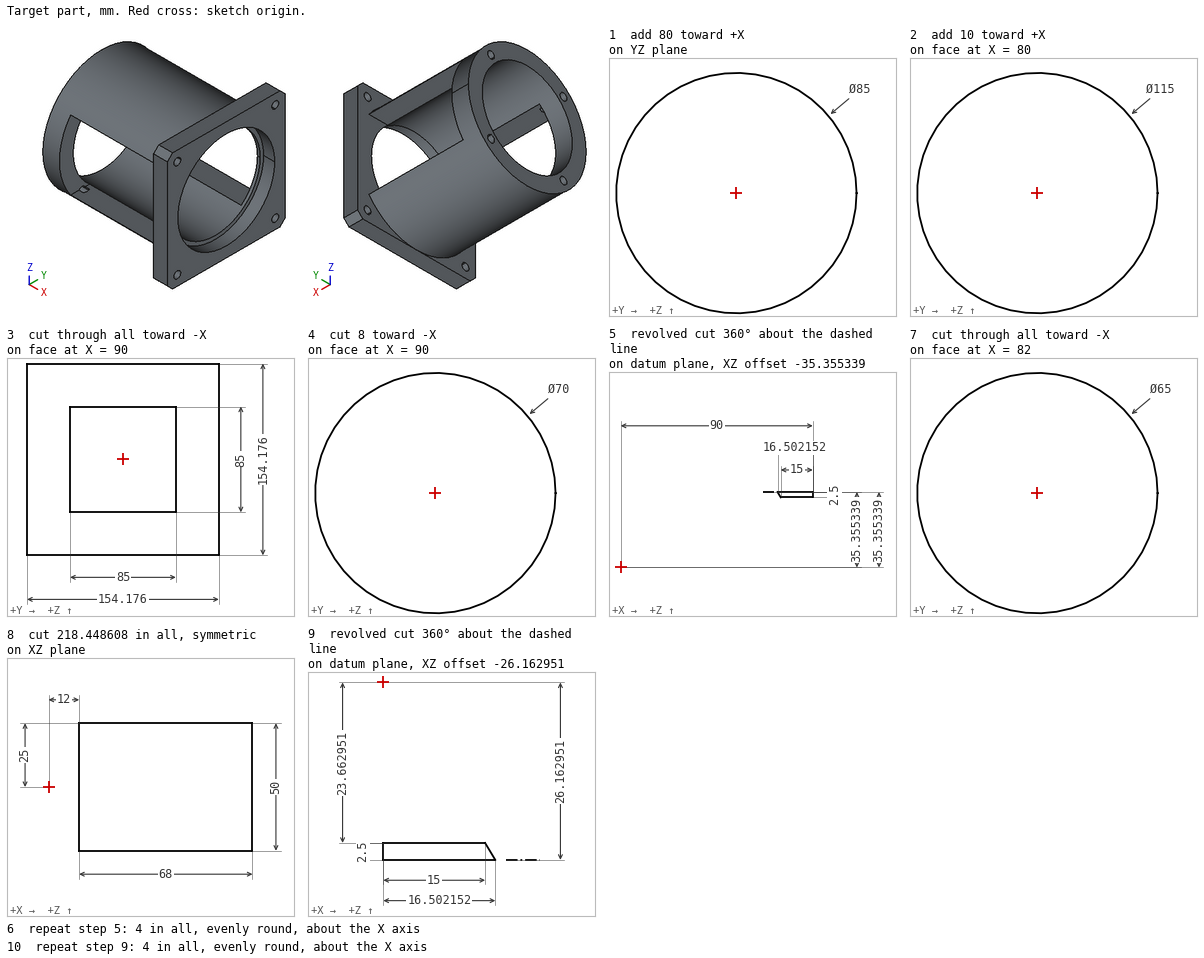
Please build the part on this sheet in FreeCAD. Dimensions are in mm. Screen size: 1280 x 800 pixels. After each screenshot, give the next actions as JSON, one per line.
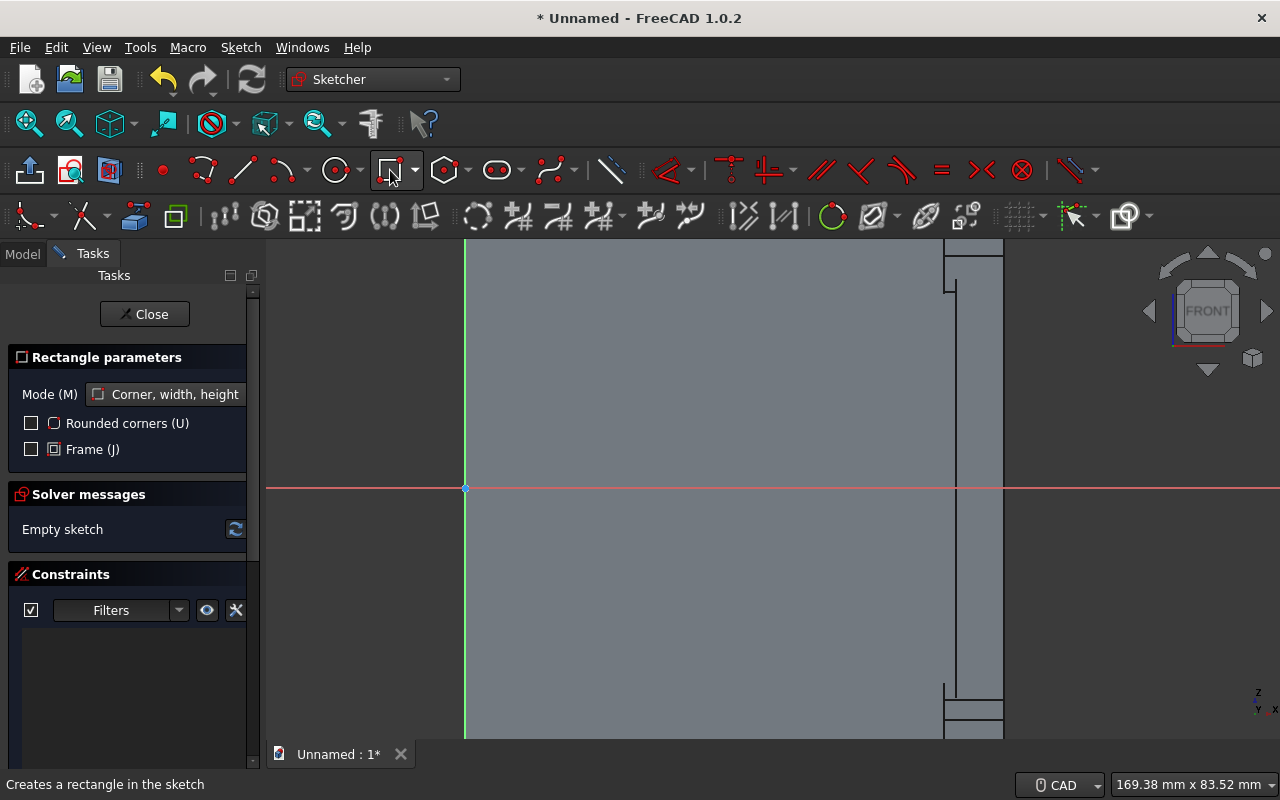
{"action": "left_click", "coordinate": [537, 339]}
{"action": "mouse_move", "coordinate": [944, 638]}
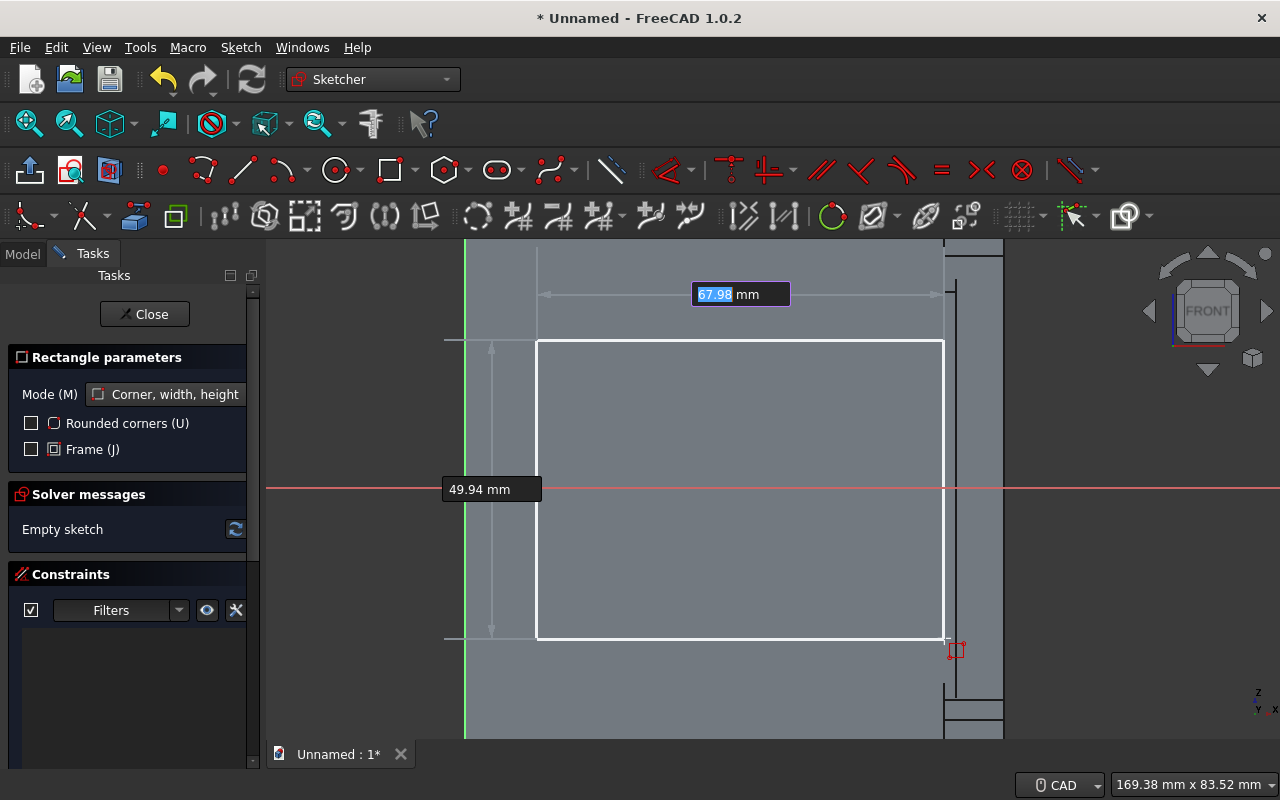
{"action": "type", "text": "68"}
{"action": "key", "text": "Tab"}
{"action": "type", "text": "50"}
{"action": "key", "text": "Return"}
{"action": "key", "text": "Escape"}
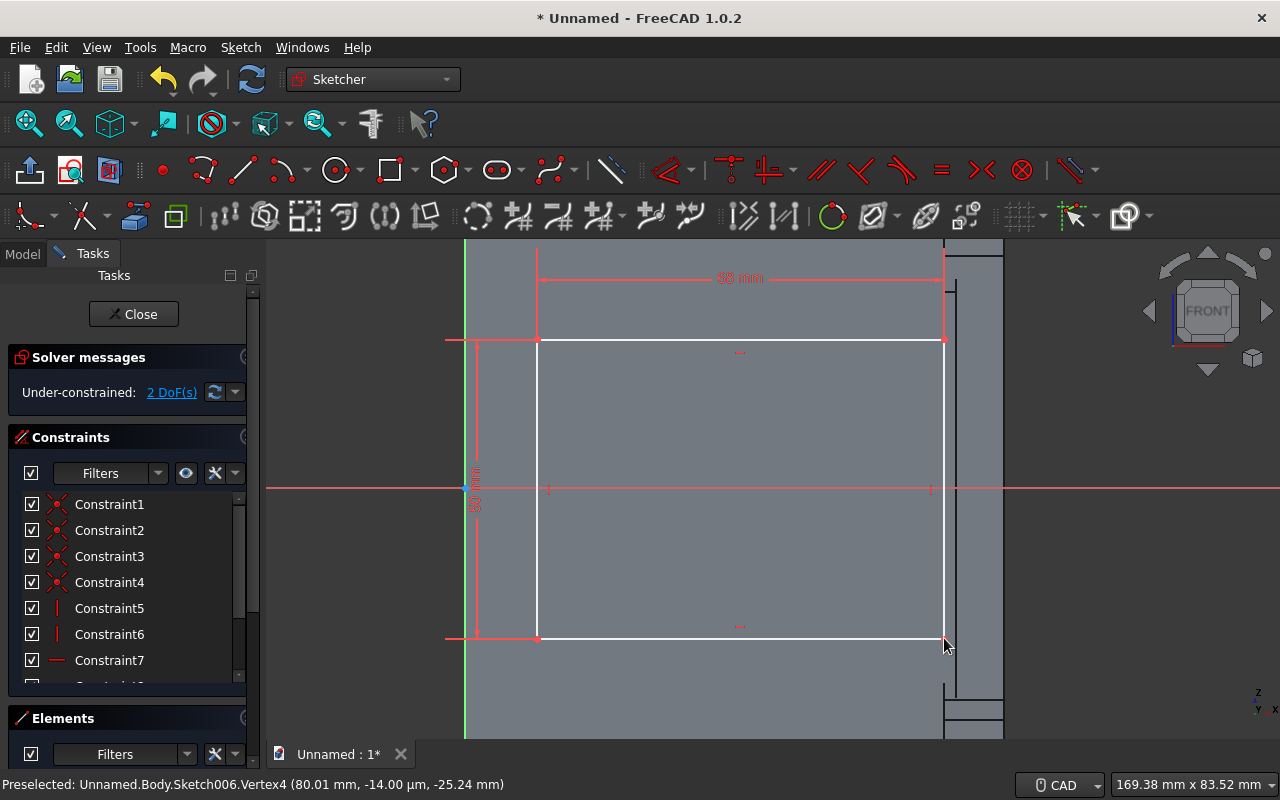
{"action": "left_click", "coordinate": [666, 170]}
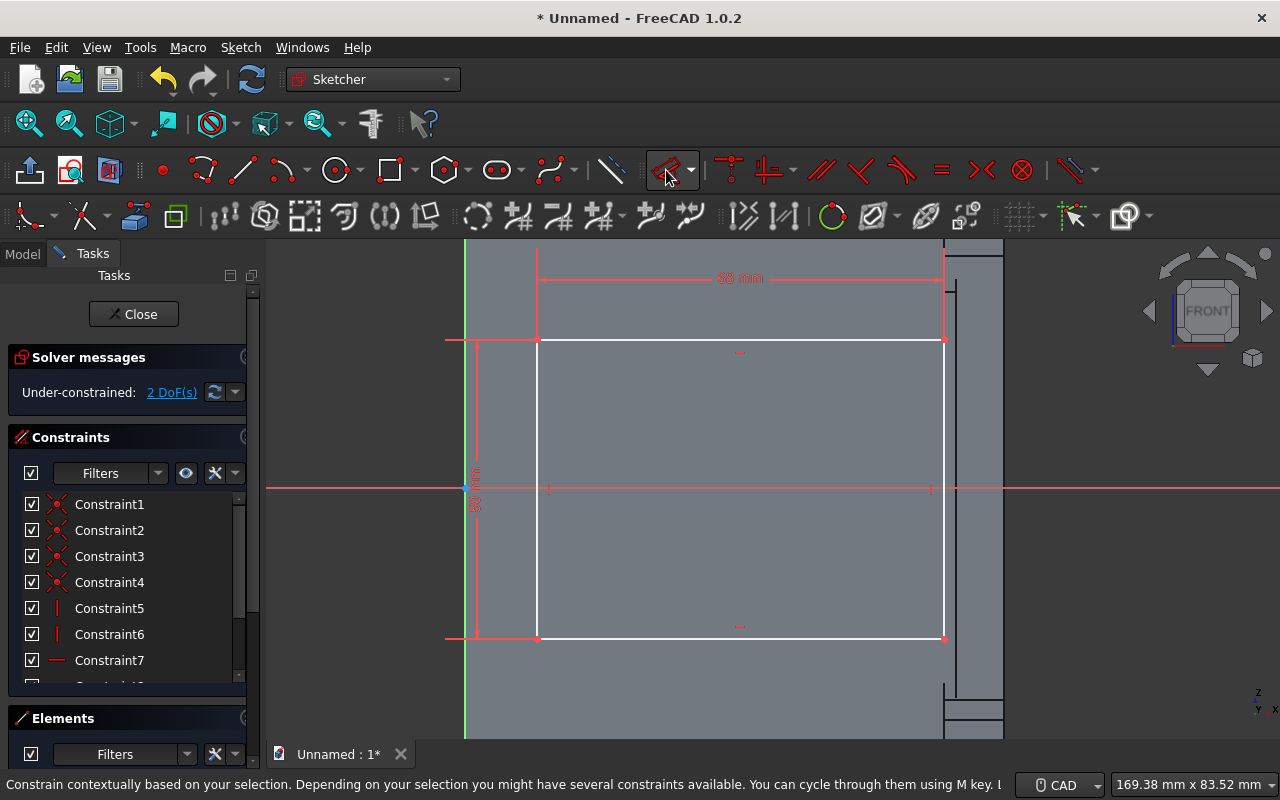
{"action": "left_click", "coordinate": [537, 340]}
{"action": "left_click", "coordinate": [501, 306]}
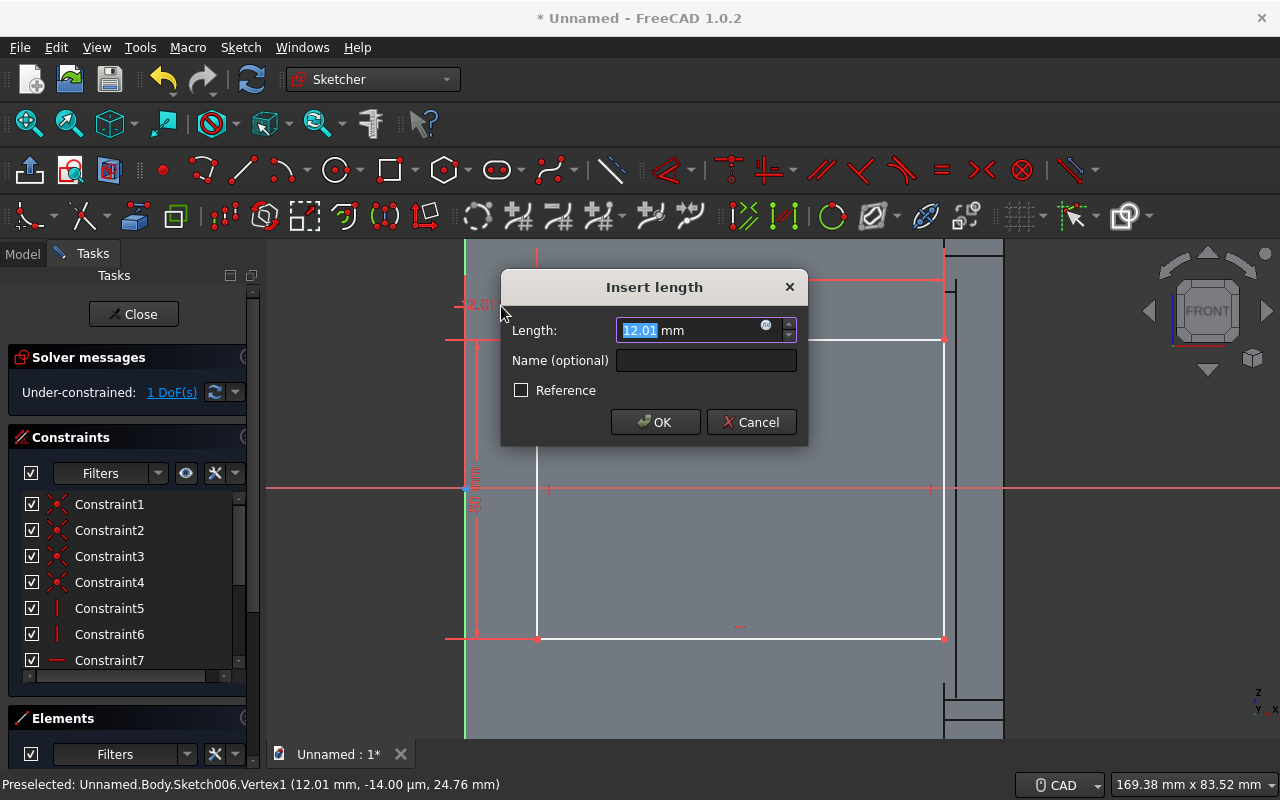
{"action": "type", "text": "12"}
{"action": "key", "text": "Return"}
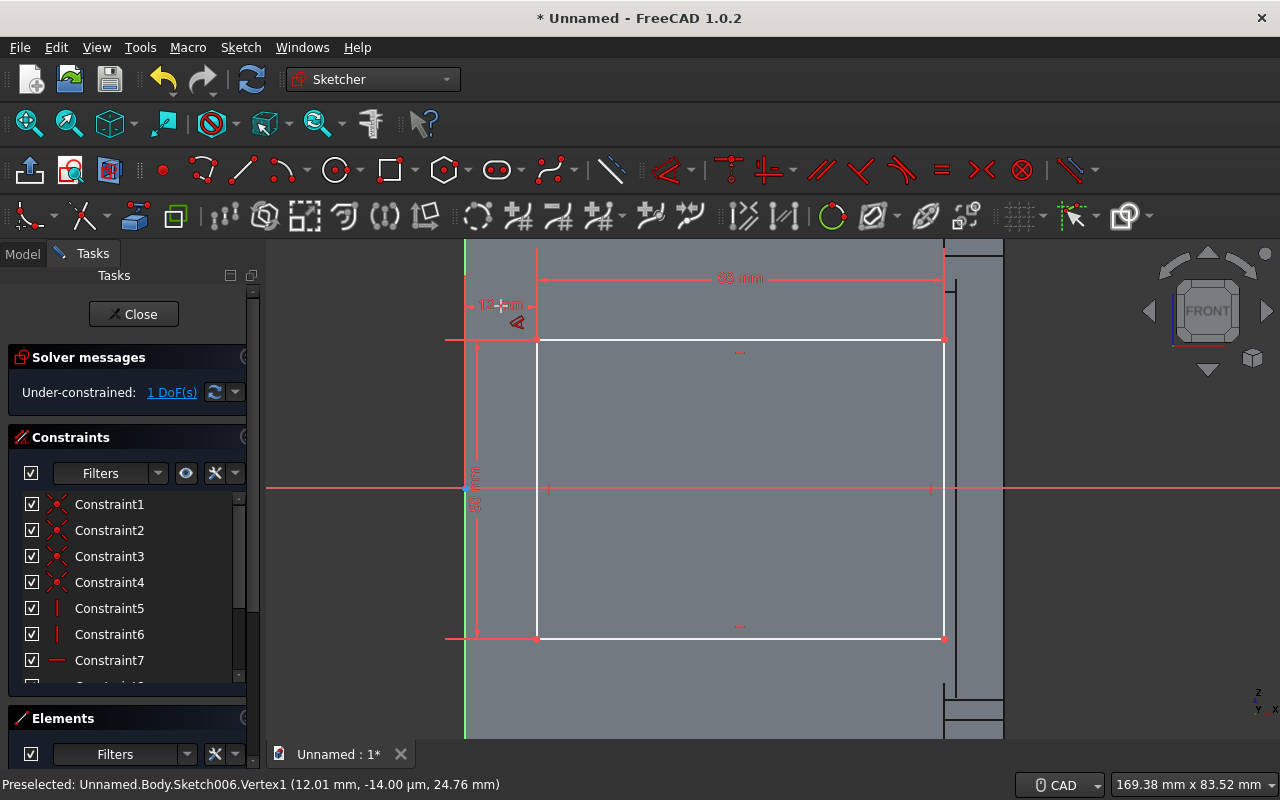
{"action": "left_click", "coordinate": [537, 340]}
{"action": "left_click", "coordinate": [431, 414]}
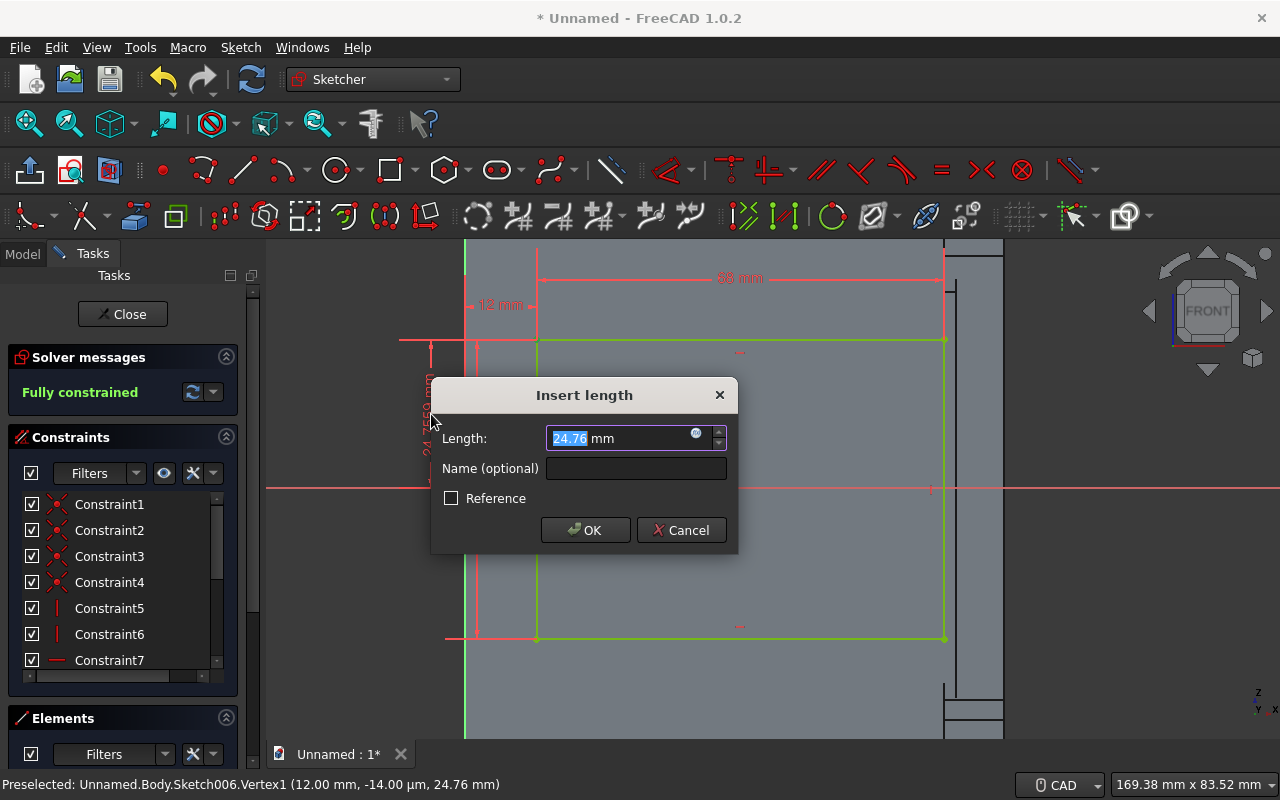
{"action": "type", "text": "25"}
{"action": "key", "text": "Return"}
{"action": "key", "text": "Escape"}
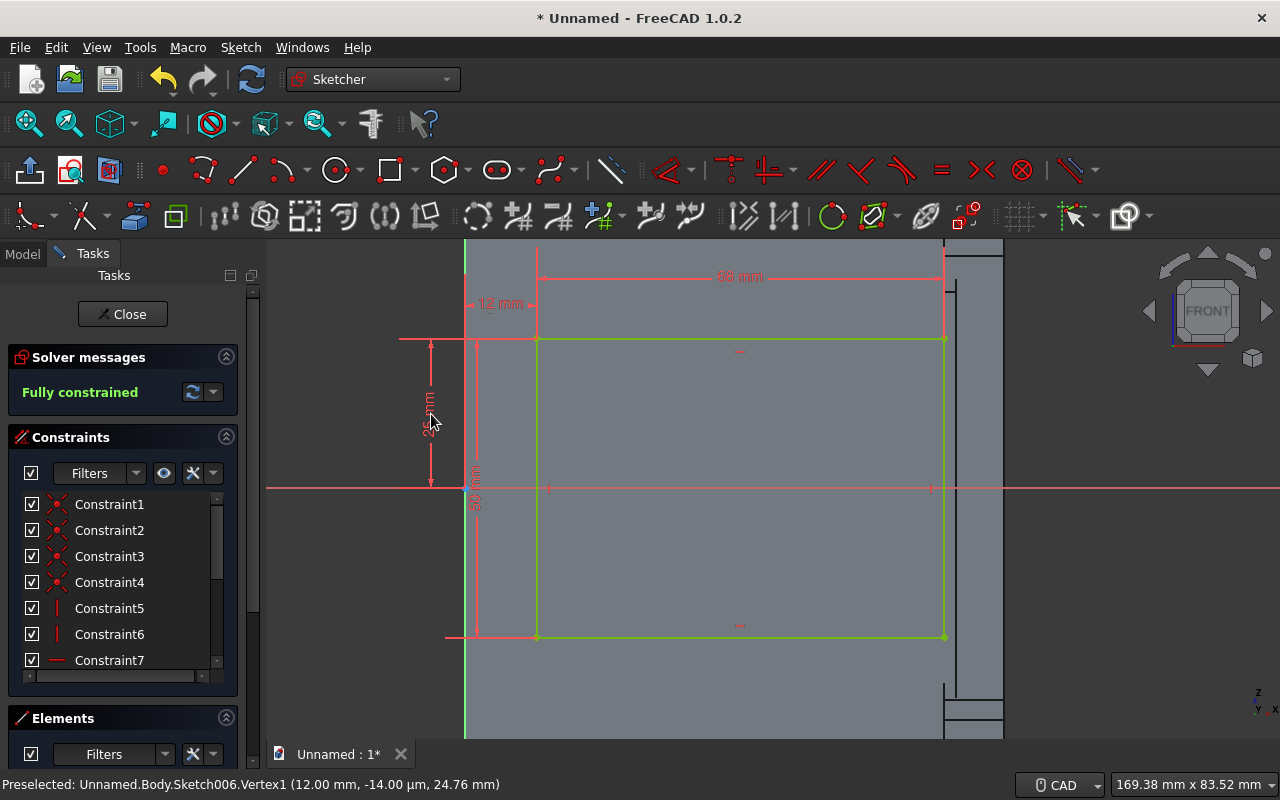
{"action": "left_click", "coordinate": [123, 314]}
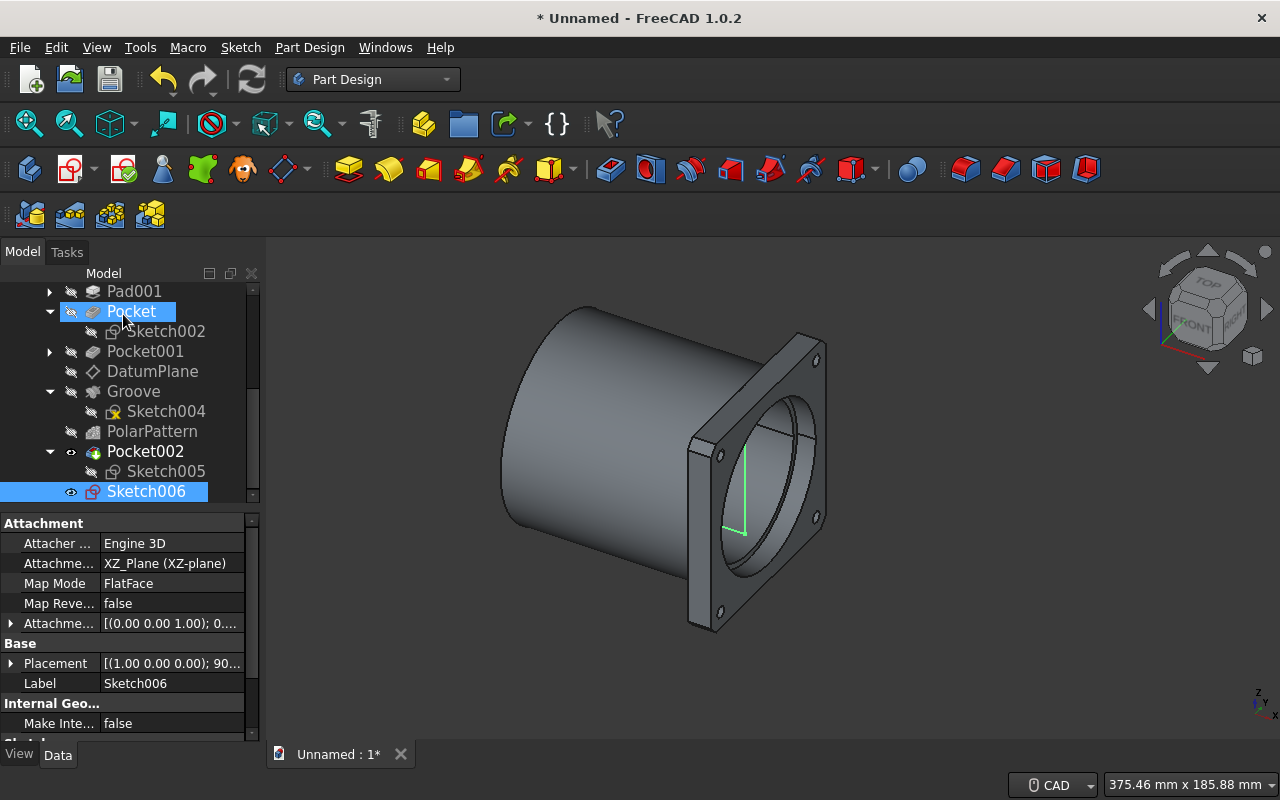
{"action": "left_click", "coordinate": [612, 170]}